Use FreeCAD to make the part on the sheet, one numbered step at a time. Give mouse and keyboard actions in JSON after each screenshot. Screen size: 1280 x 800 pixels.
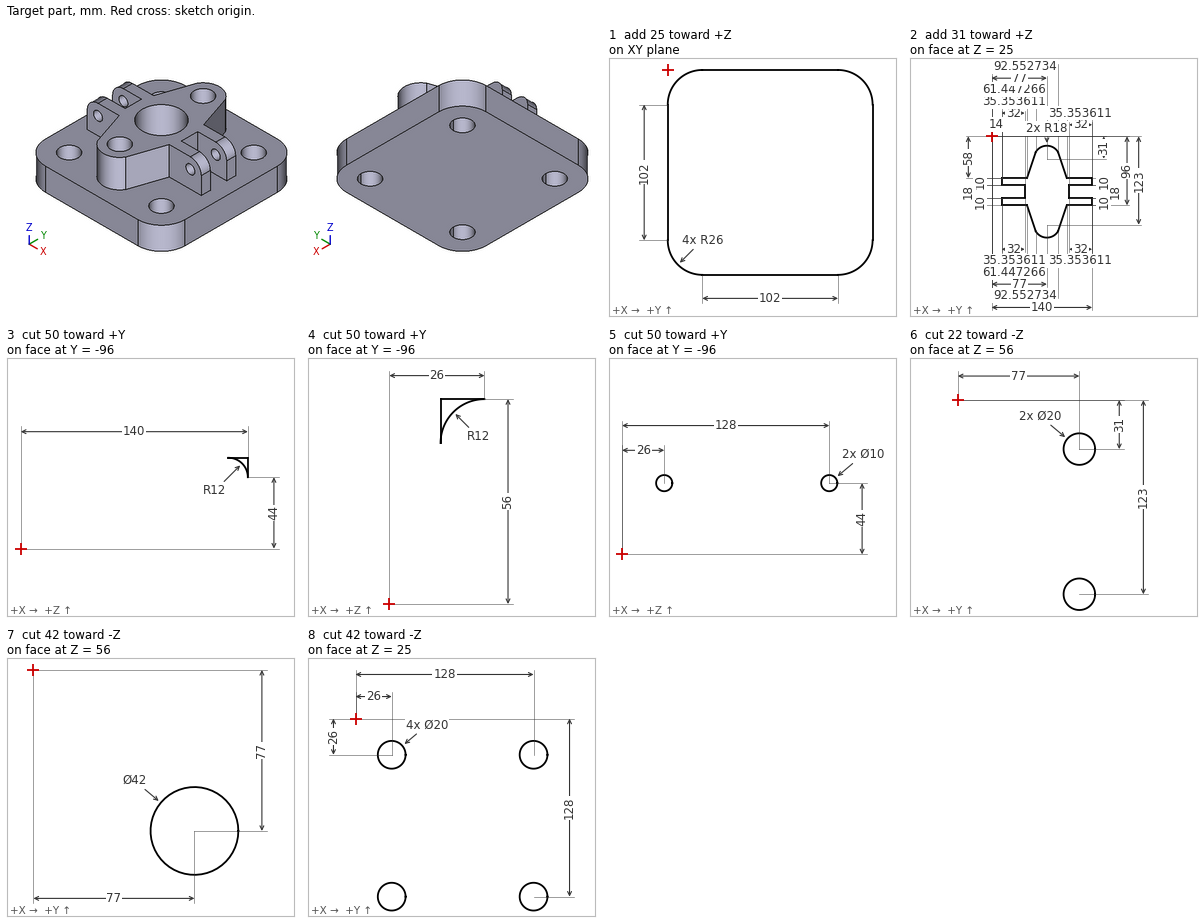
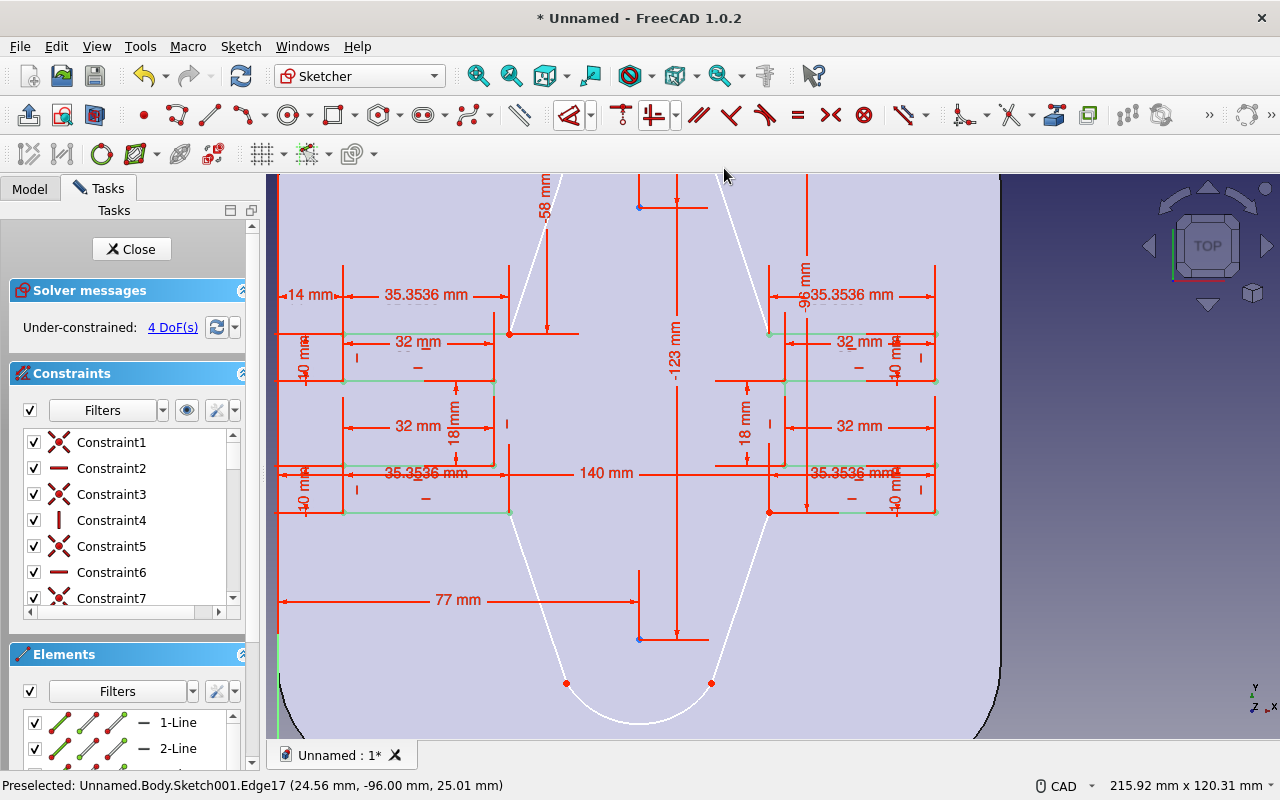
{"action": "left_click", "coordinate": [712, 683]}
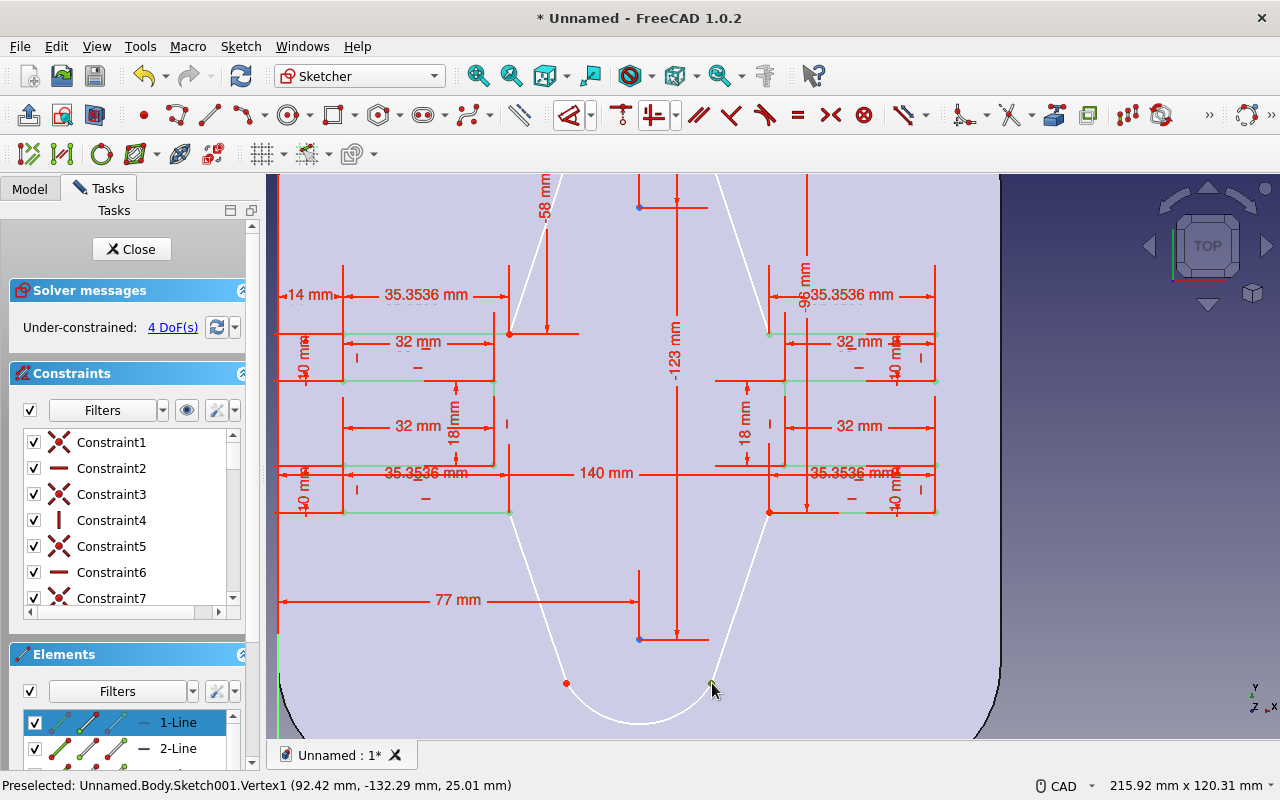
{"action": "left_click", "coordinate": [590, 116]}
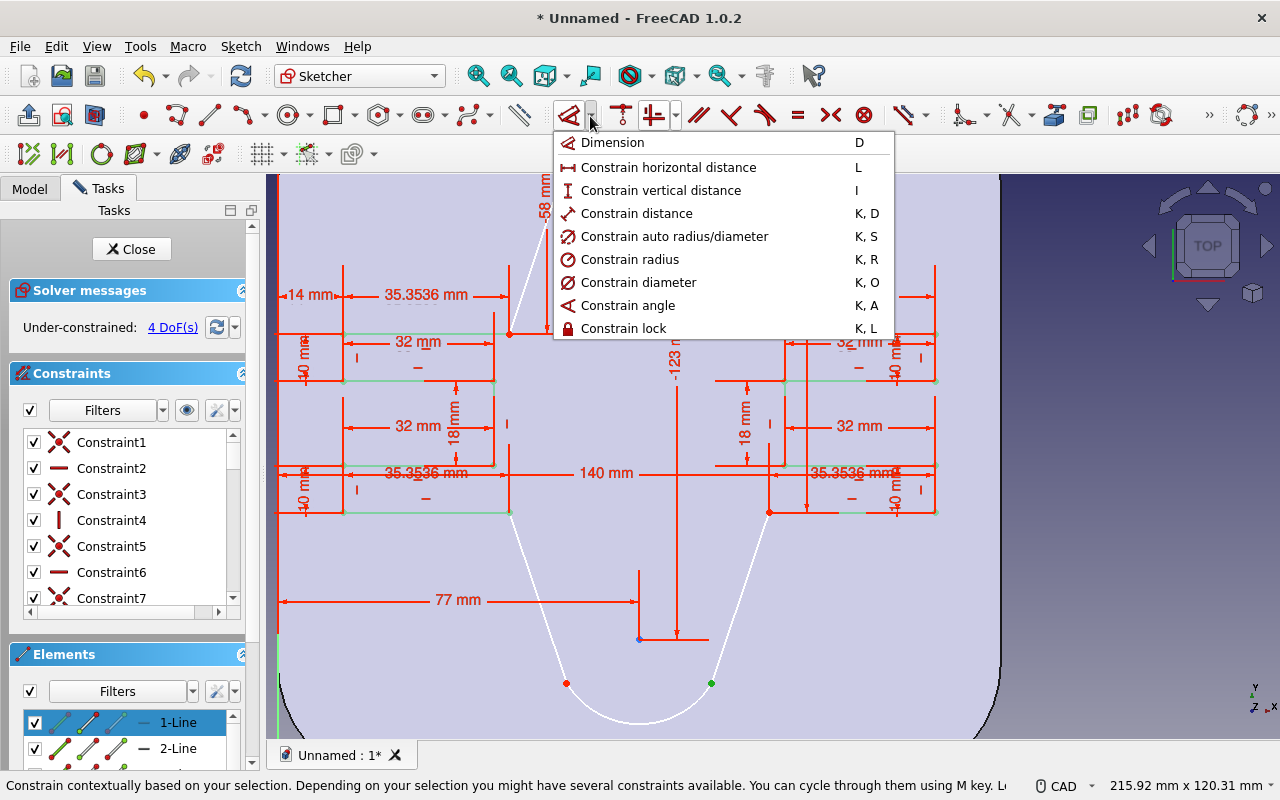
{"action": "left_click", "coordinate": [724, 168]}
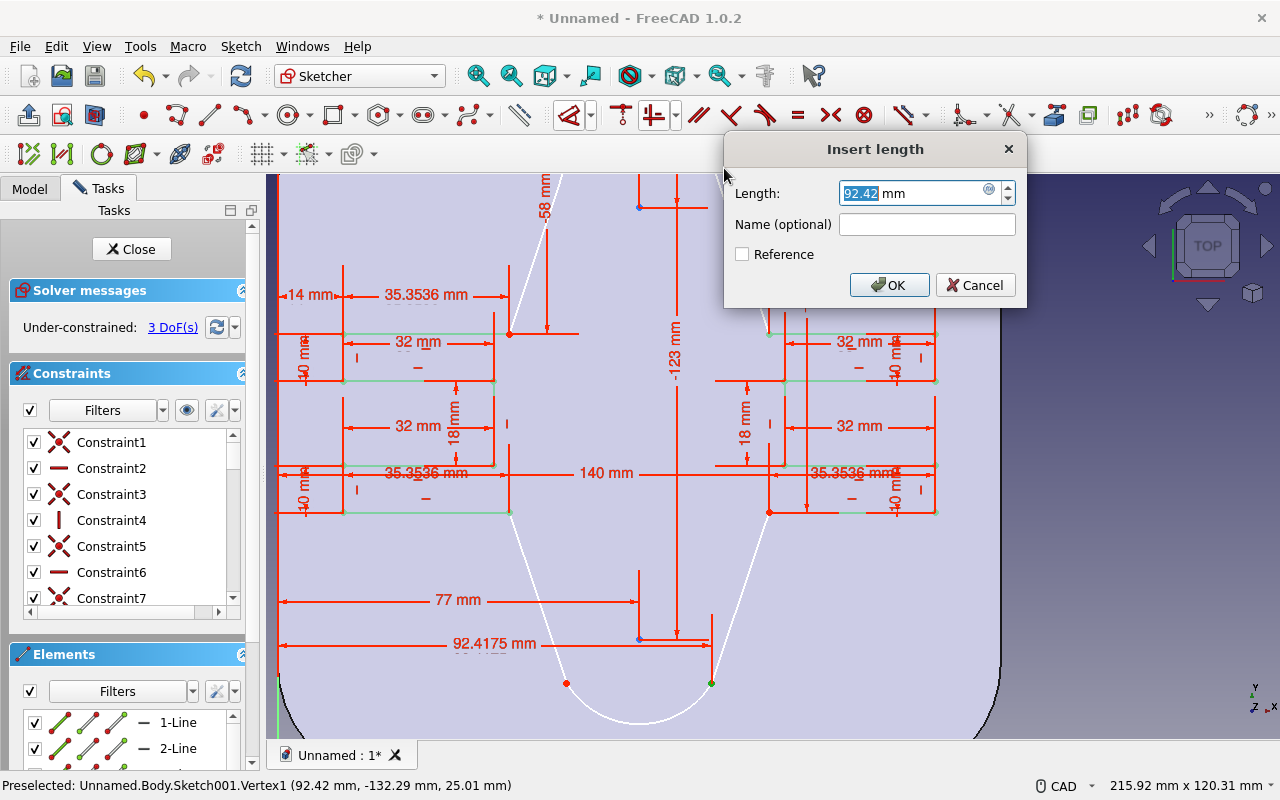
{"action": "type", "text": "92.552734"}
{"action": "key", "text": "Return"}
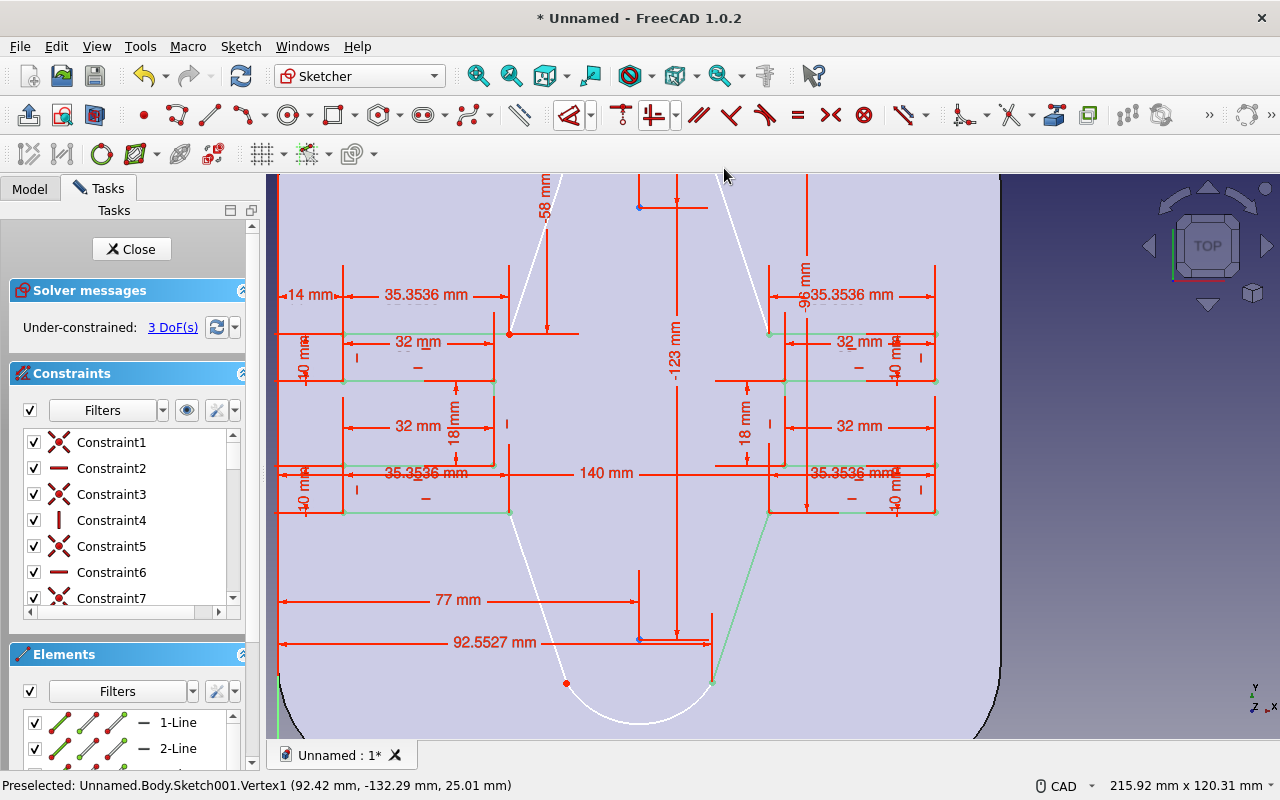
{"action": "scroll", "coordinate": [824, 534], "scroll_direction": "down", "scroll_amount": 3}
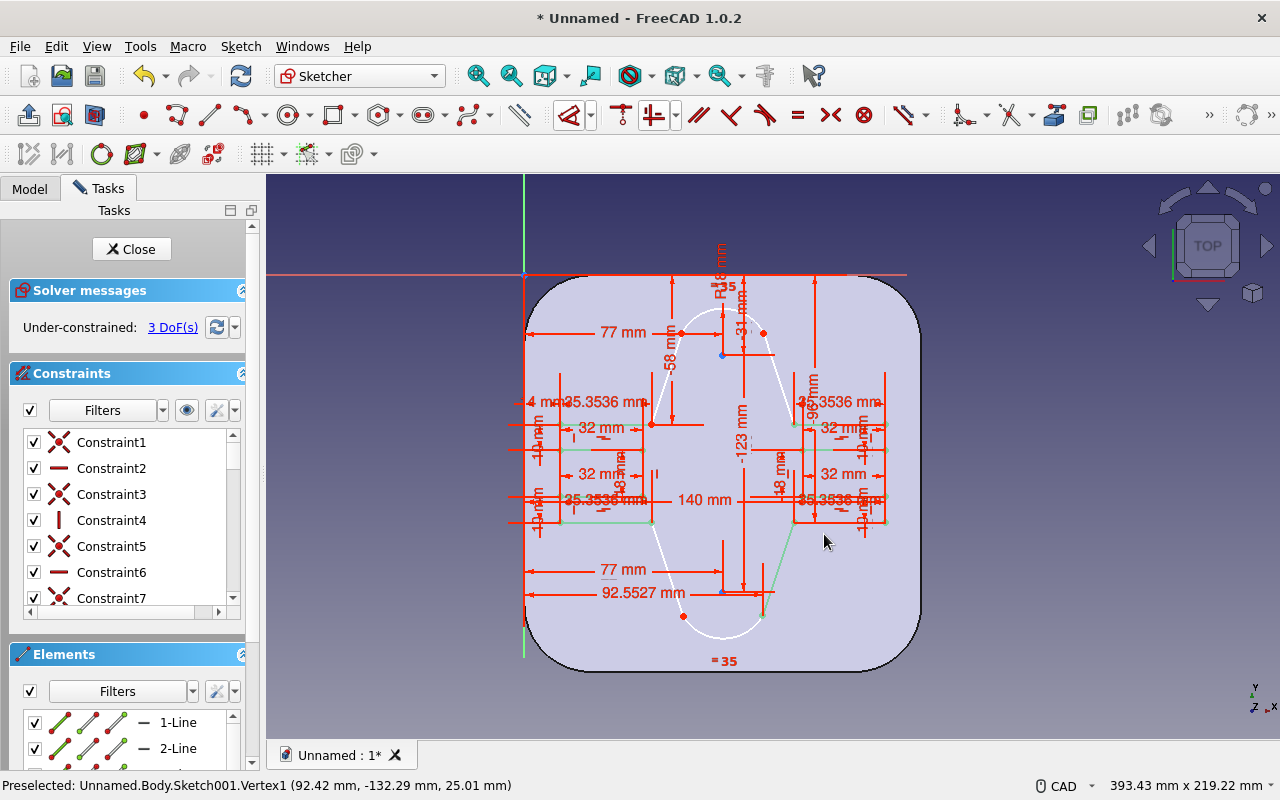
{"action": "left_click", "coordinate": [764, 333]}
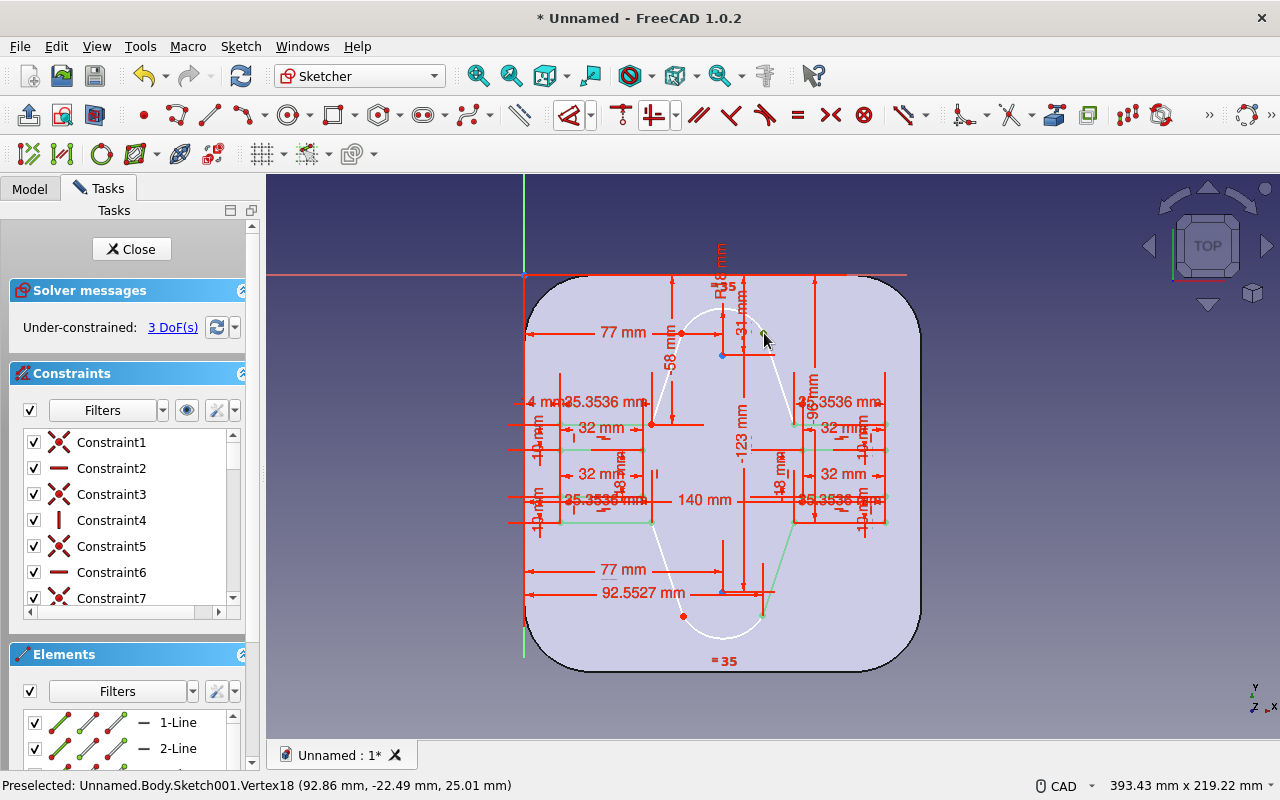
{"action": "key", "text": "l"}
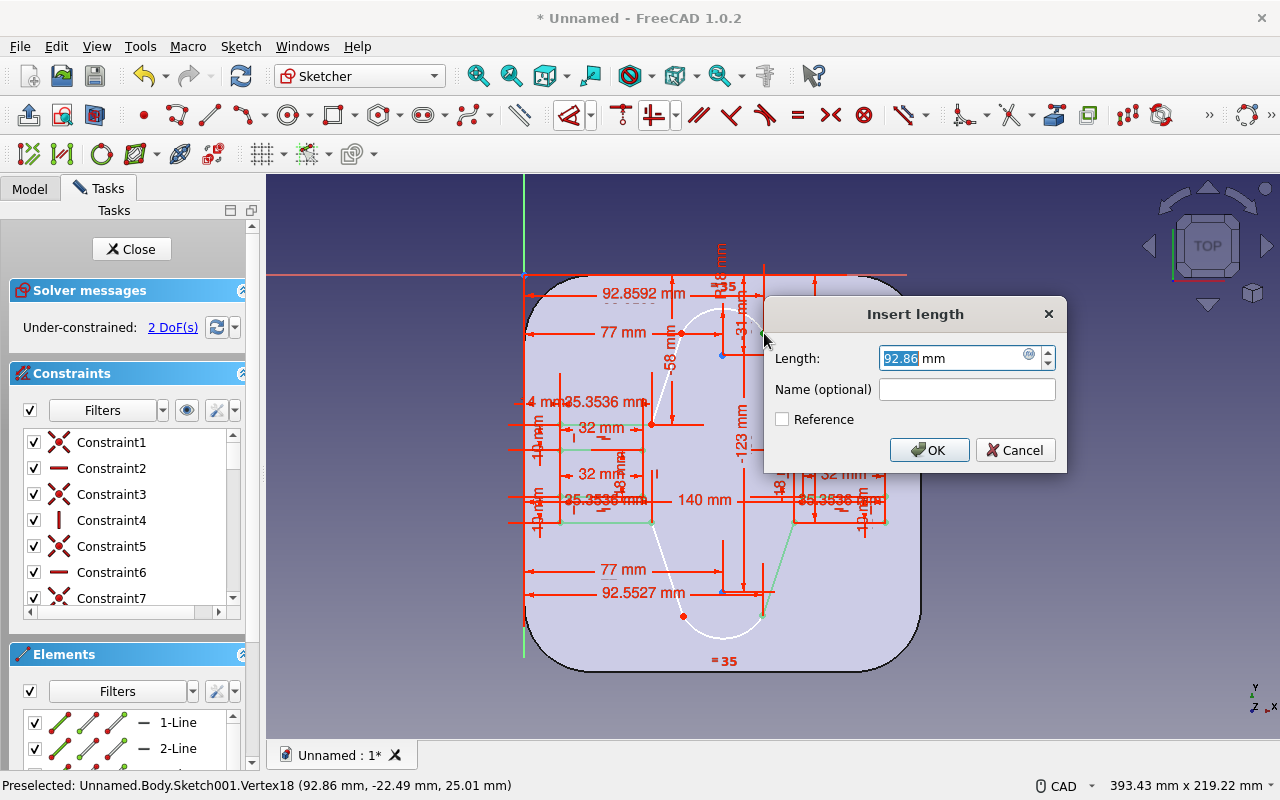
{"action": "type", "text": "92.552734"}
{"action": "key", "text": "Return"}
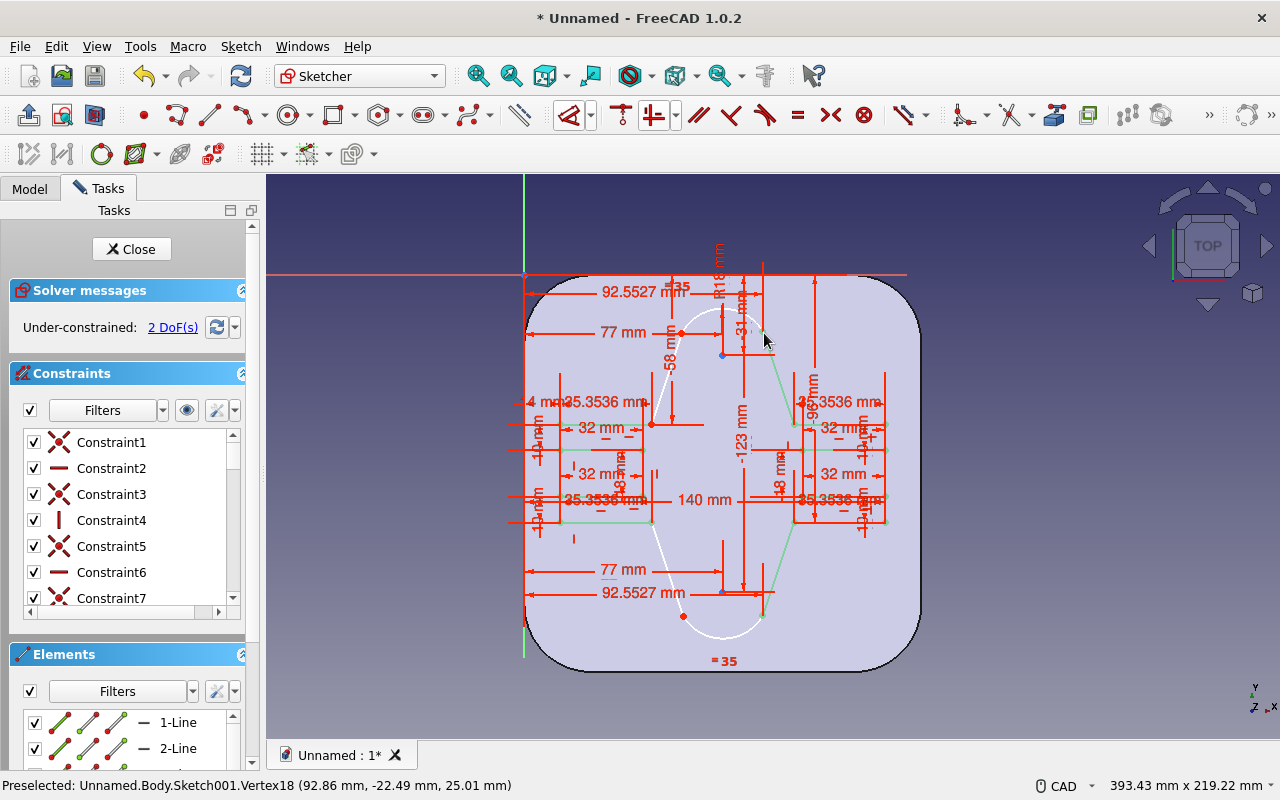
{"action": "left_click", "coordinate": [682, 333]}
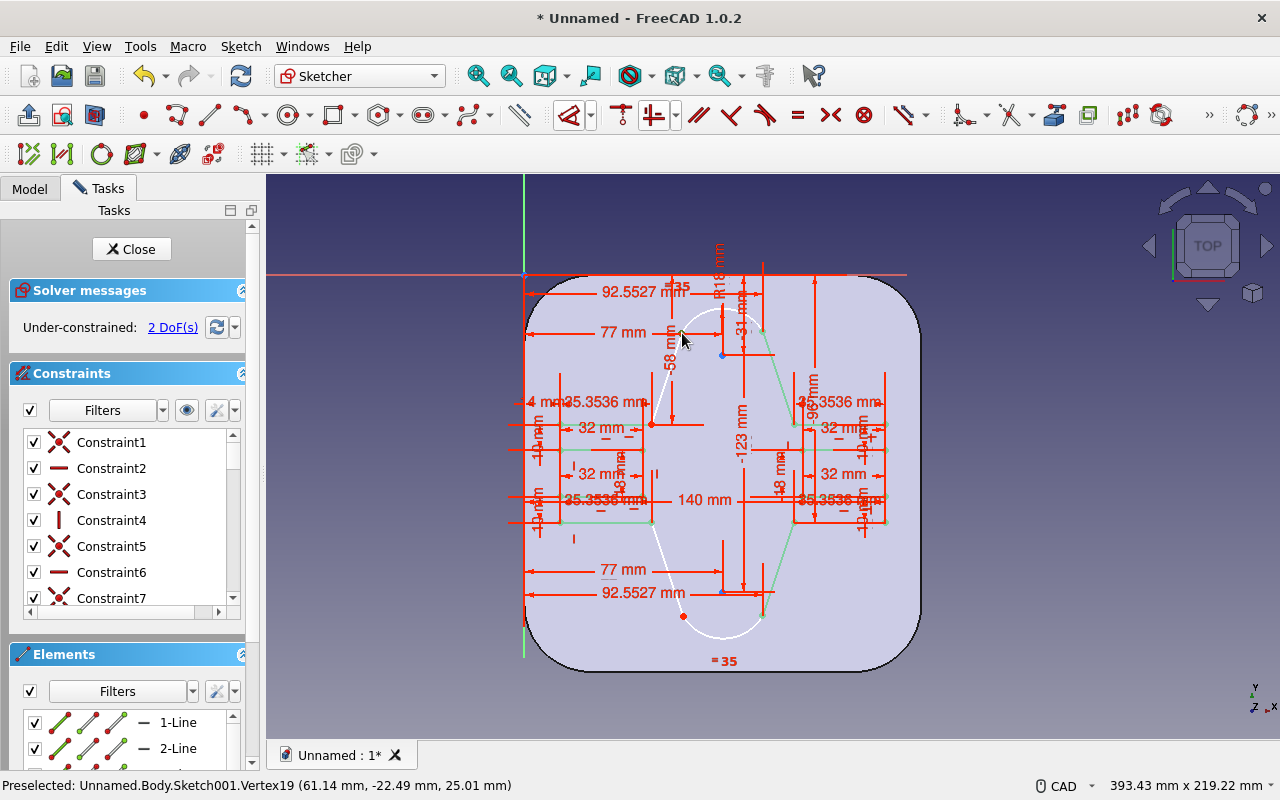
{"action": "key", "text": "l"}